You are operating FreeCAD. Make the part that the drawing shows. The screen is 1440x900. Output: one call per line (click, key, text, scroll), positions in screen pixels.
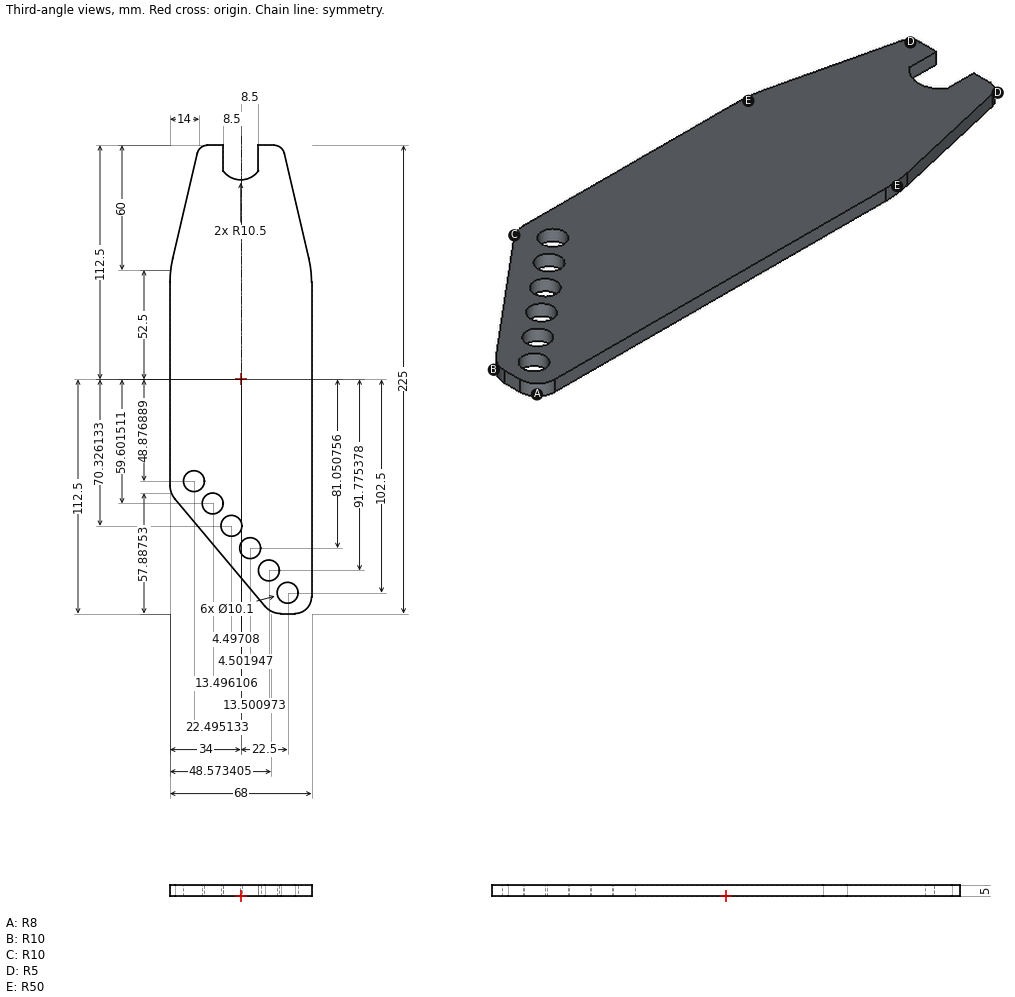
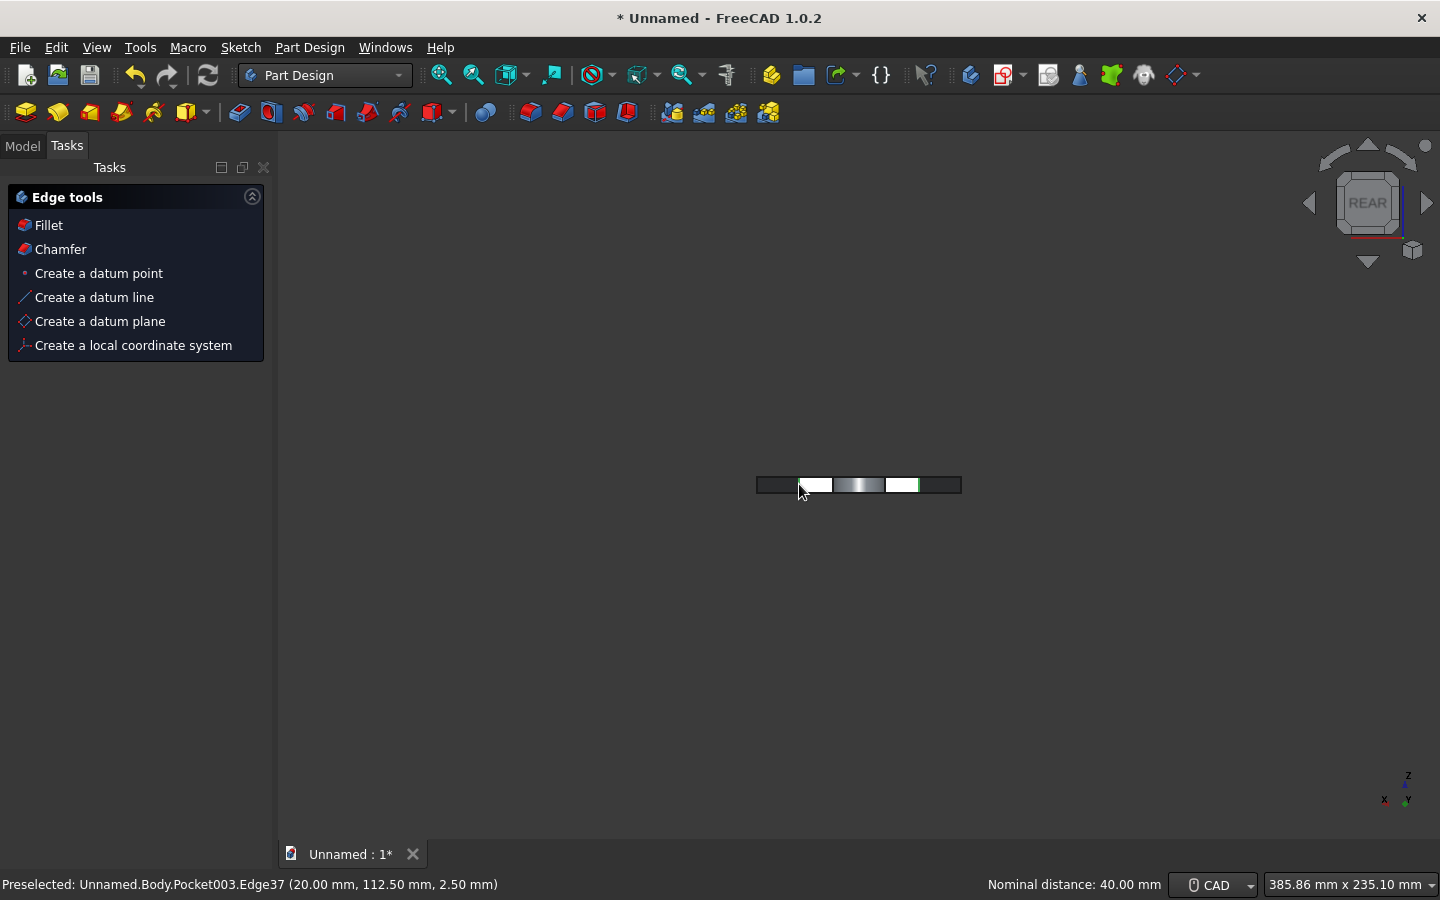
click(532, 112)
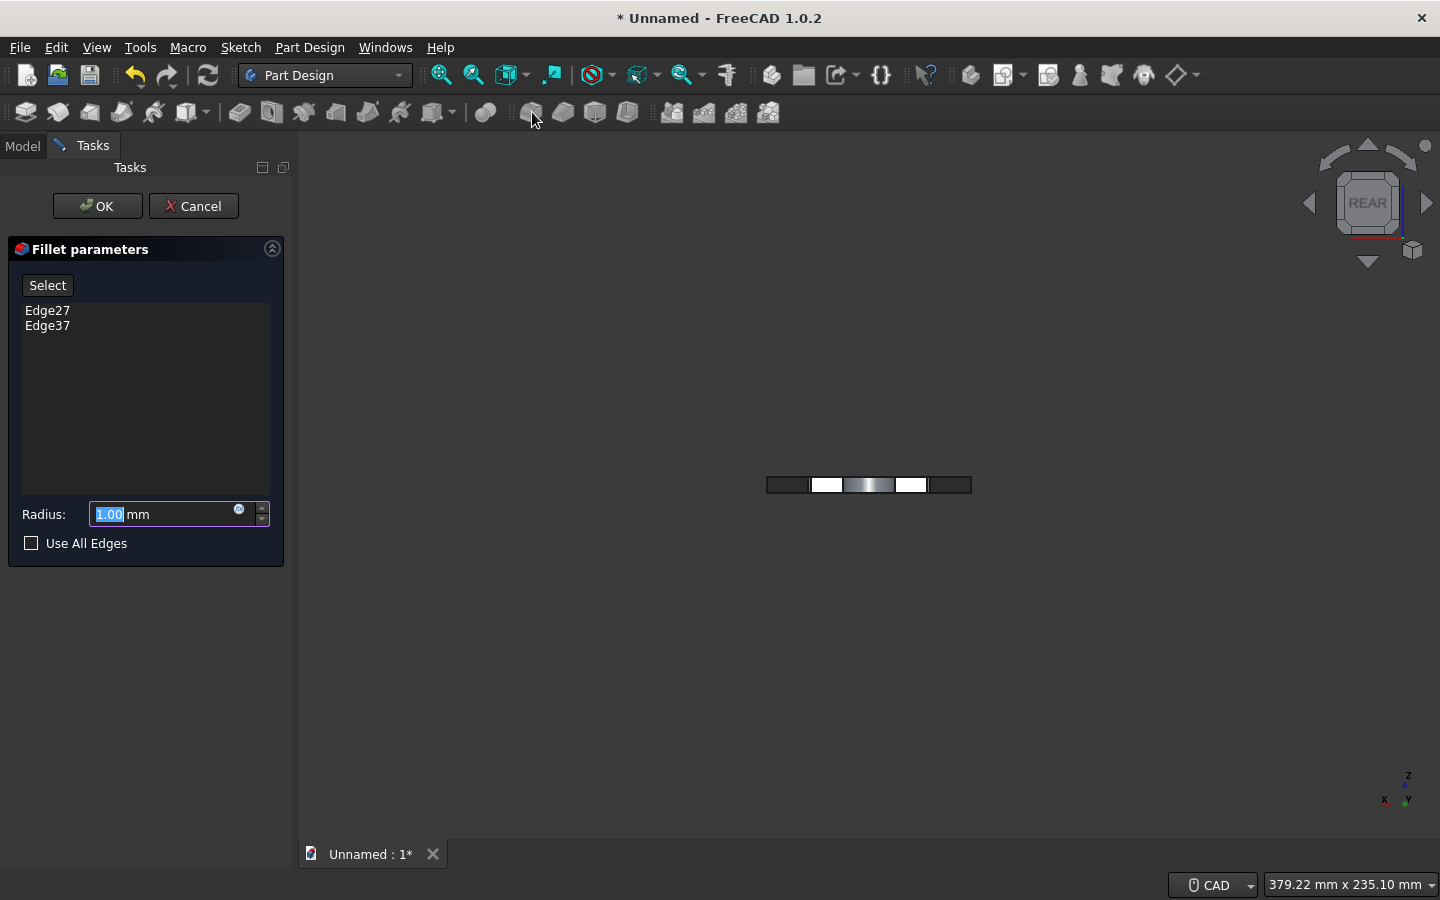
text(5)
key(Tab)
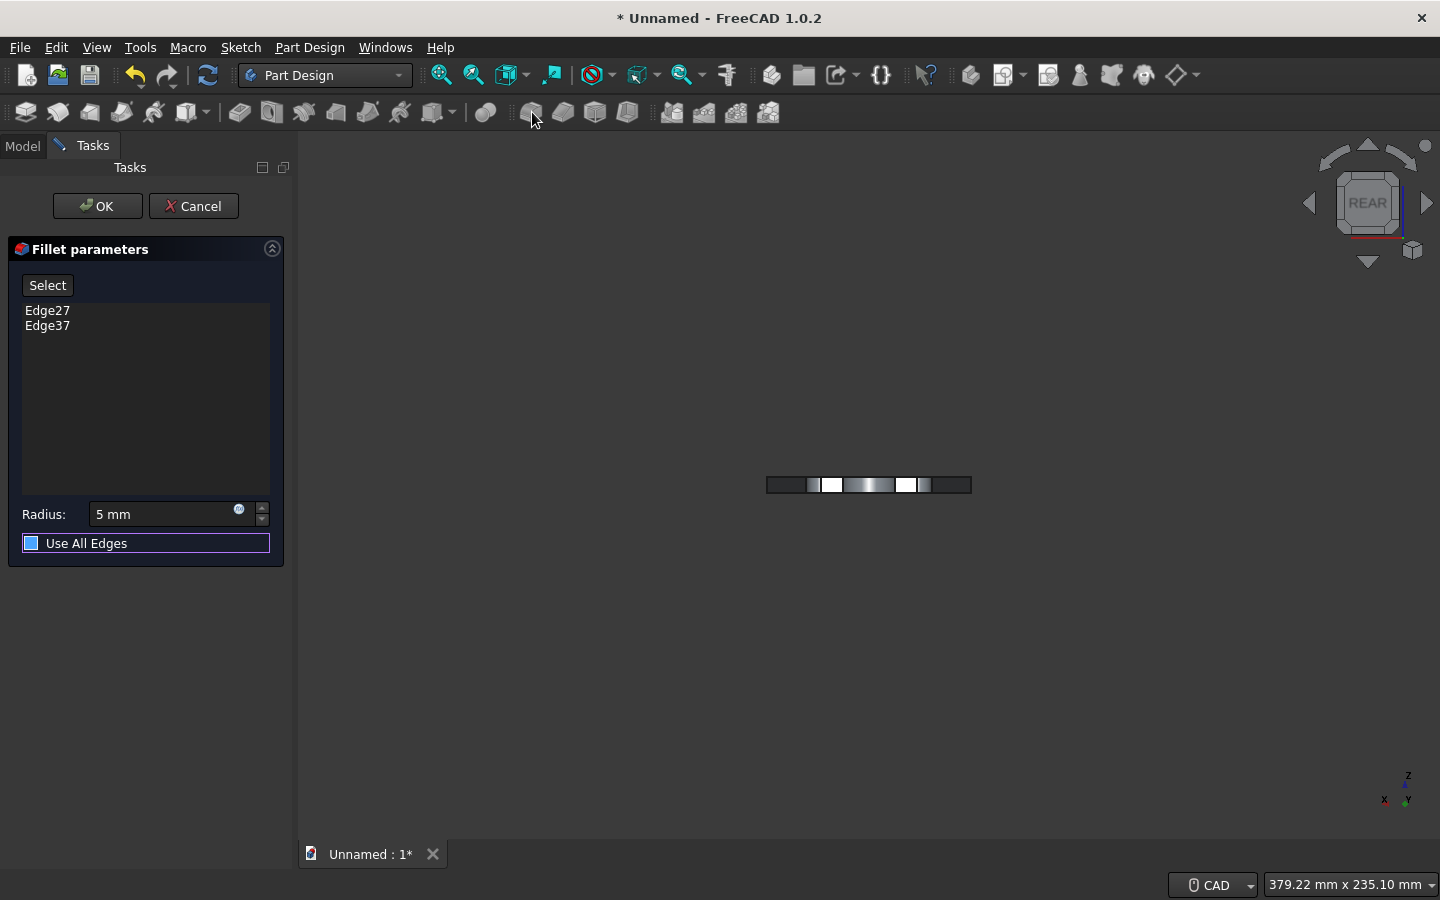
click(98, 206)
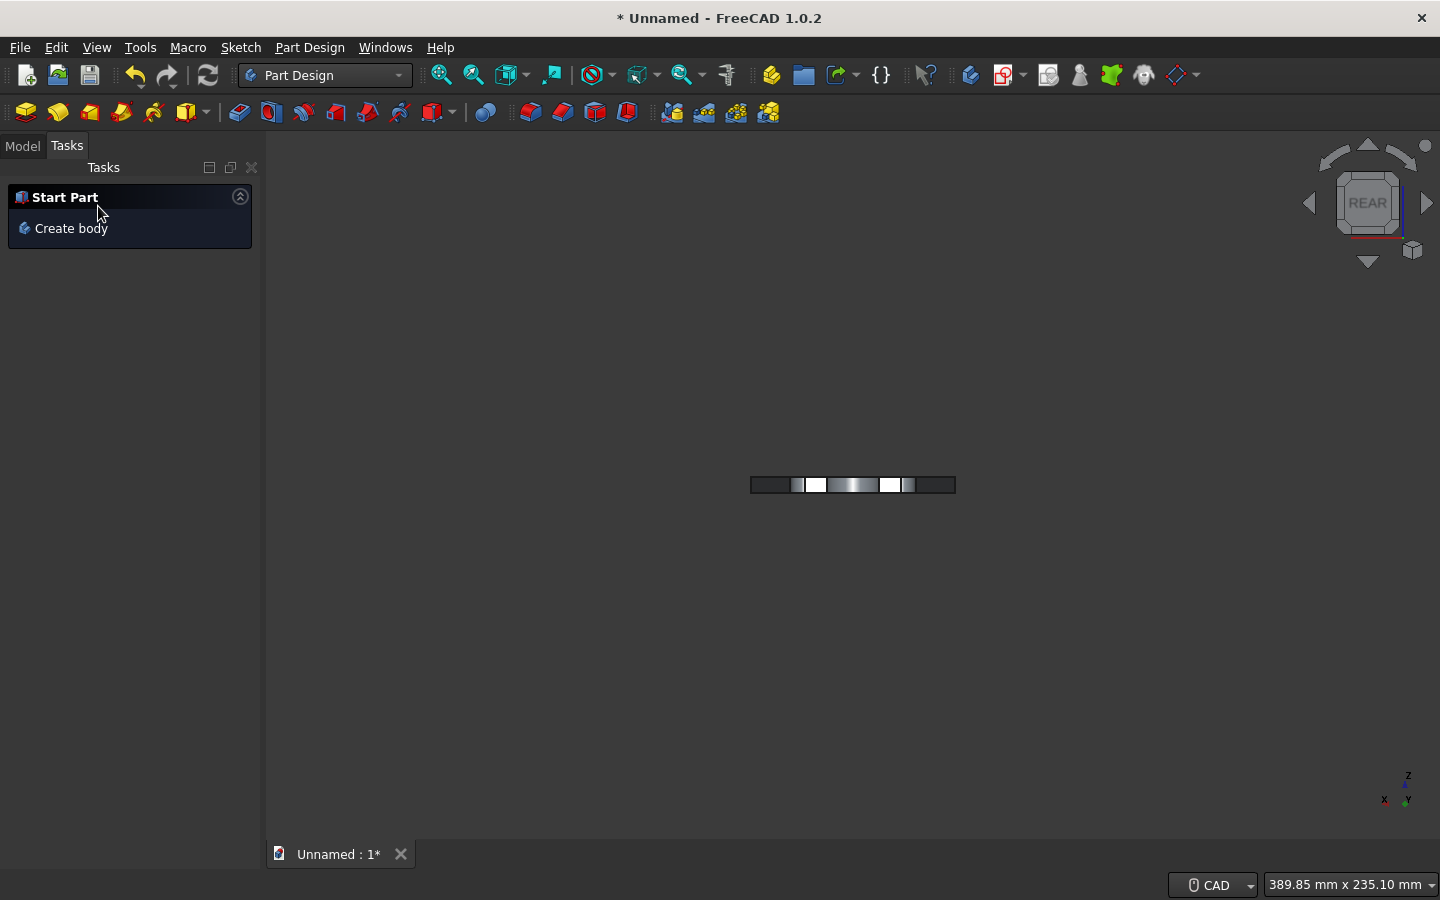
key(v)
key(f)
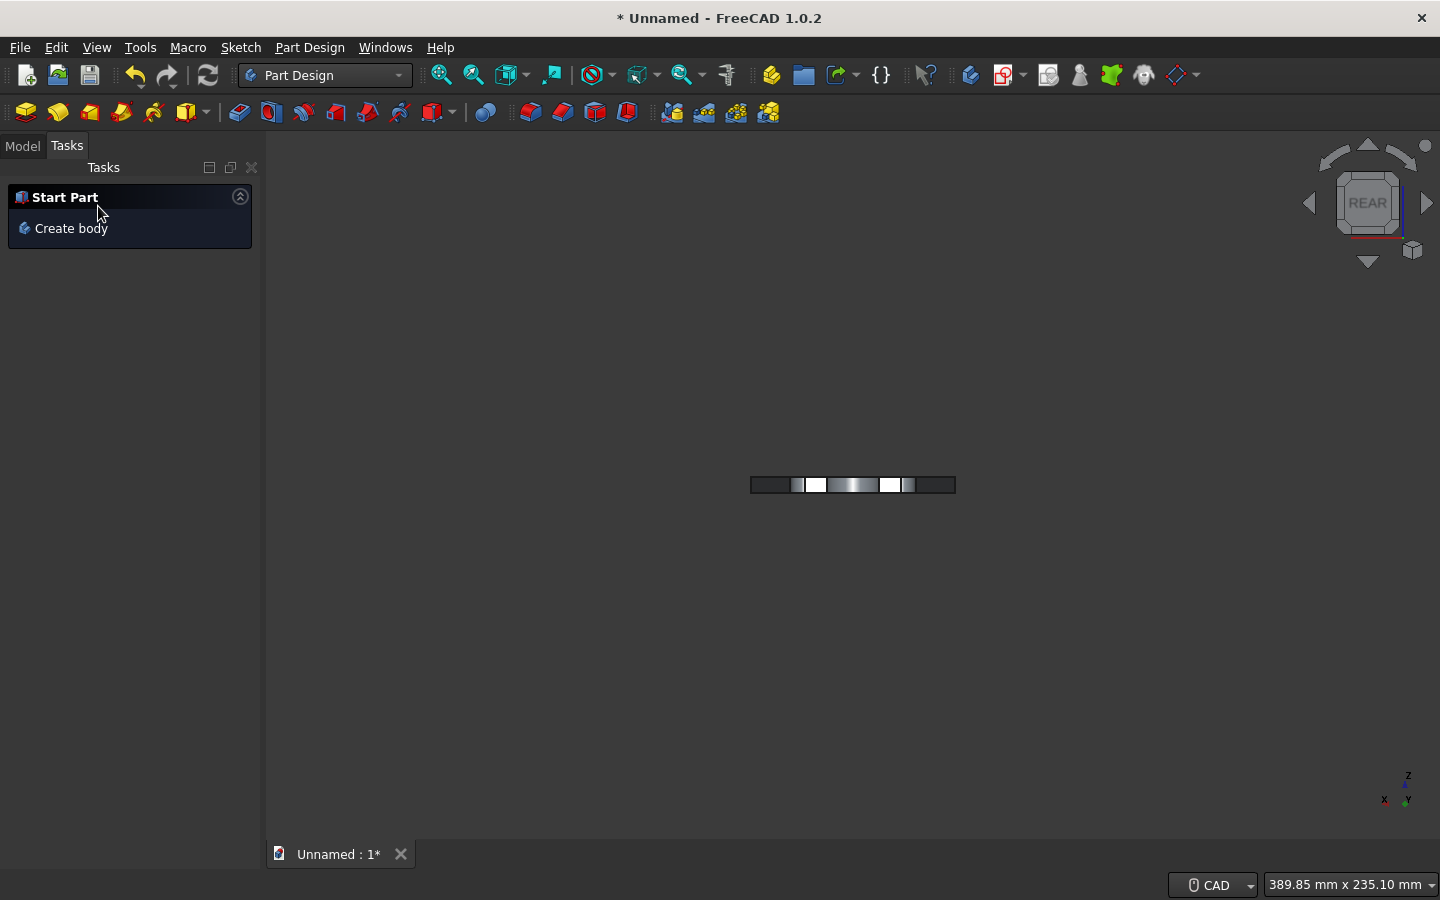
scroll(955, 484, up, 5)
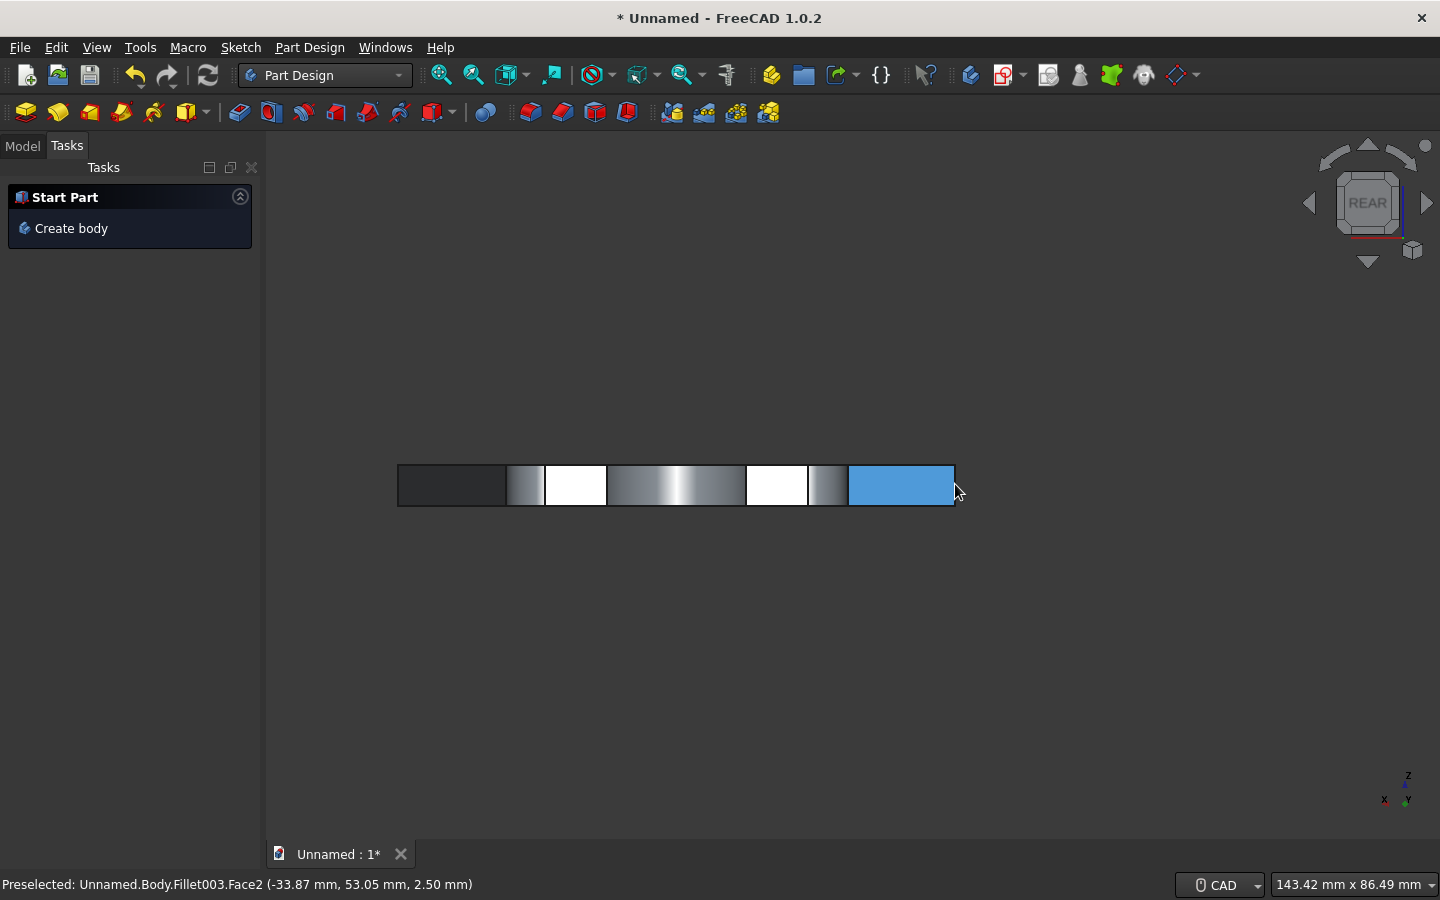
key(v)
key(f)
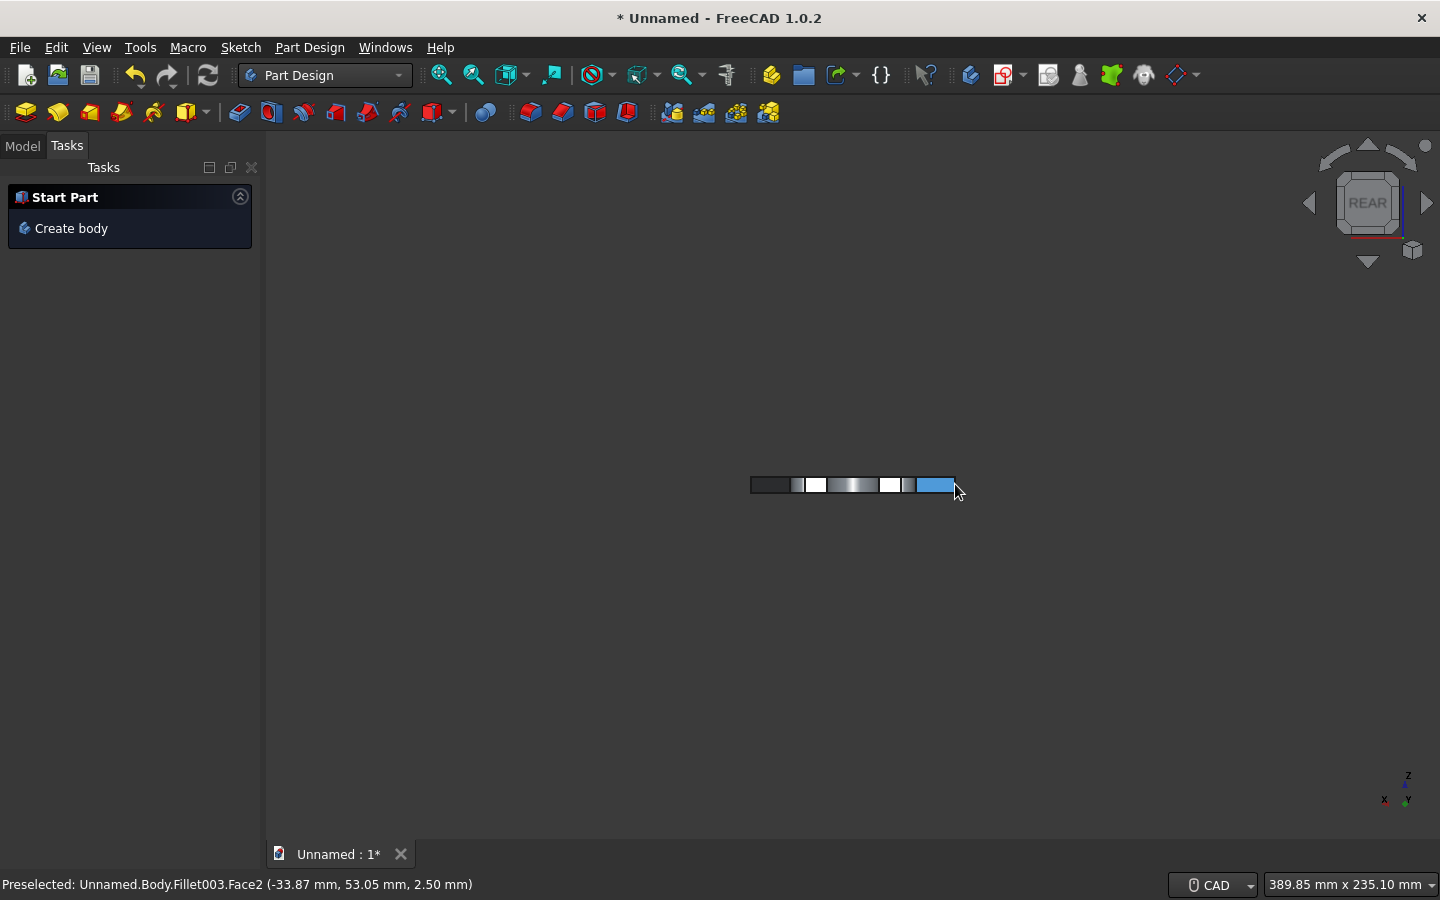
key(0)